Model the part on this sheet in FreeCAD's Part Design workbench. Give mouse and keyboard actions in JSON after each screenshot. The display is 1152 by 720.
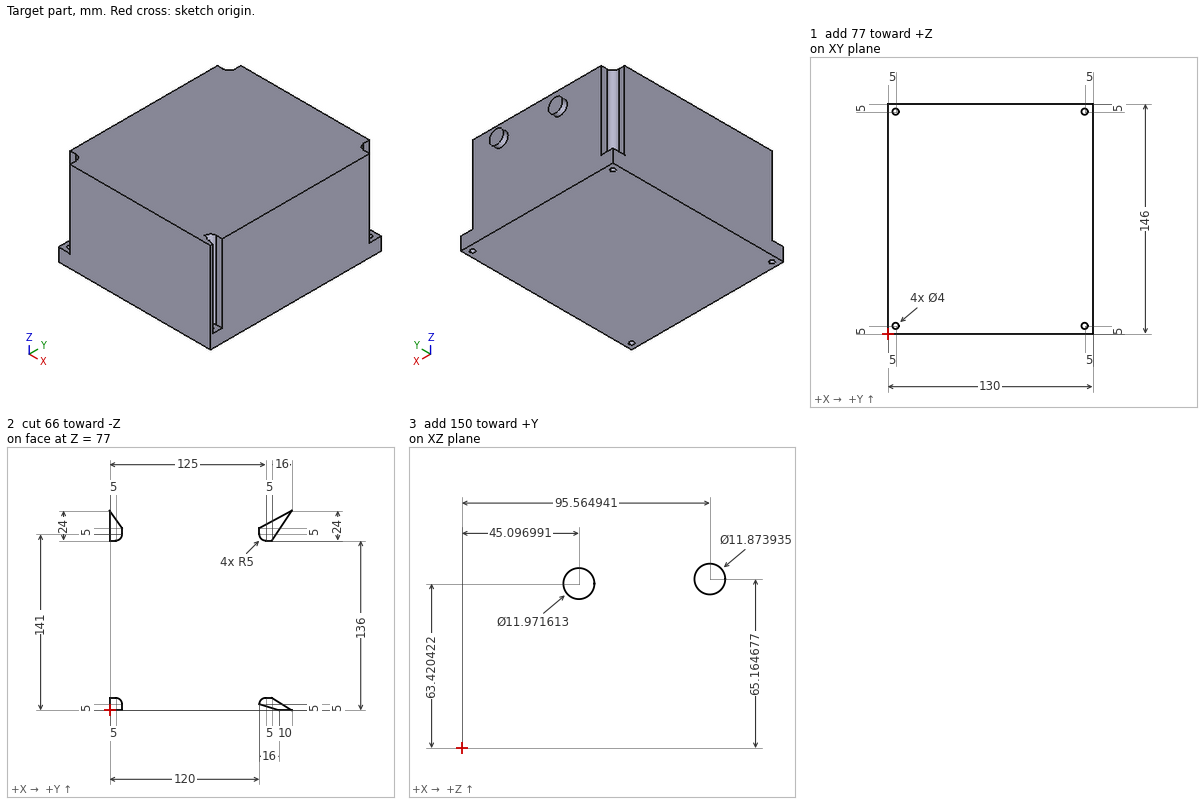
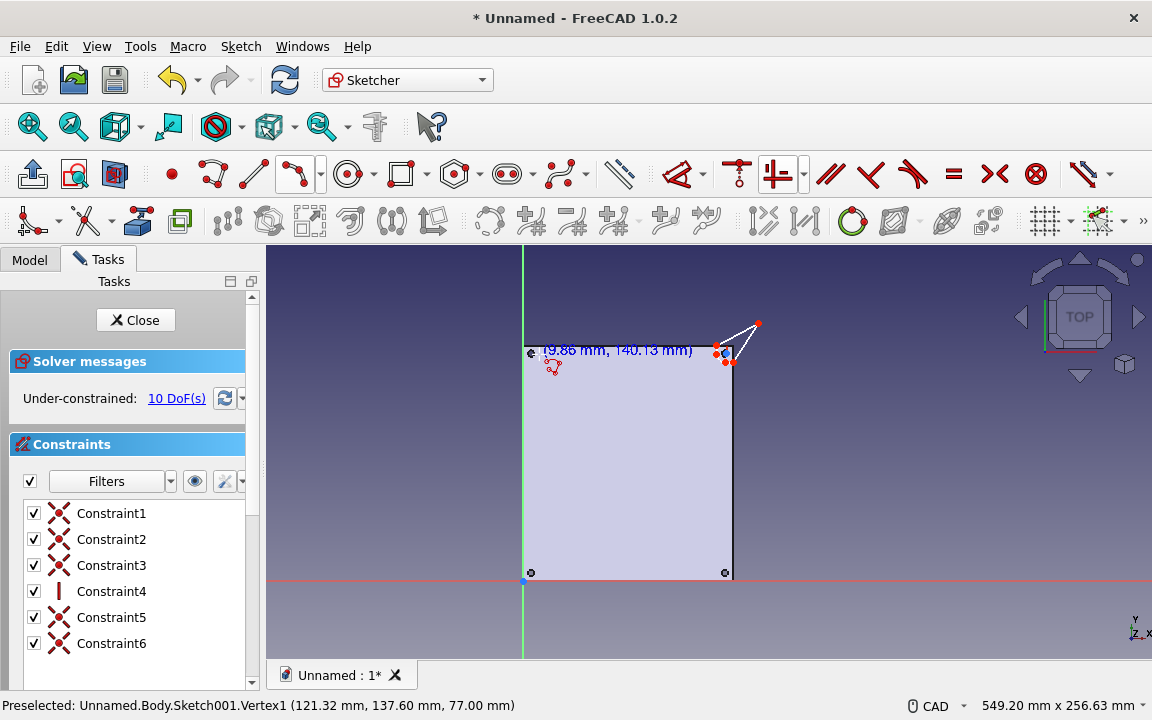
{"action": "scroll", "coordinate": [539, 346], "scroll_direction": "up", "scroll_amount": 4}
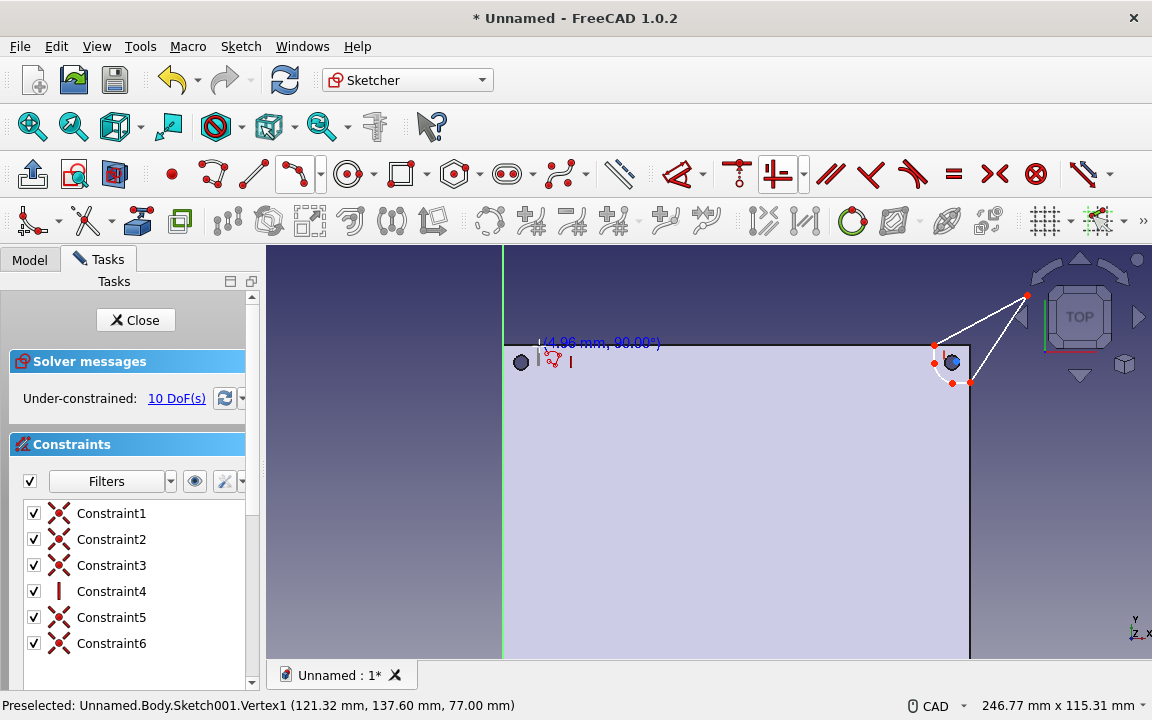
{"action": "left_click", "coordinate": [539, 345]}
{"action": "left_click", "coordinate": [503, 294]}
{"action": "left_click", "coordinate": [512, 381]}
{"action": "left_click", "coordinate": [521, 381]}
{"action": "right_click", "coordinate": [521, 381]}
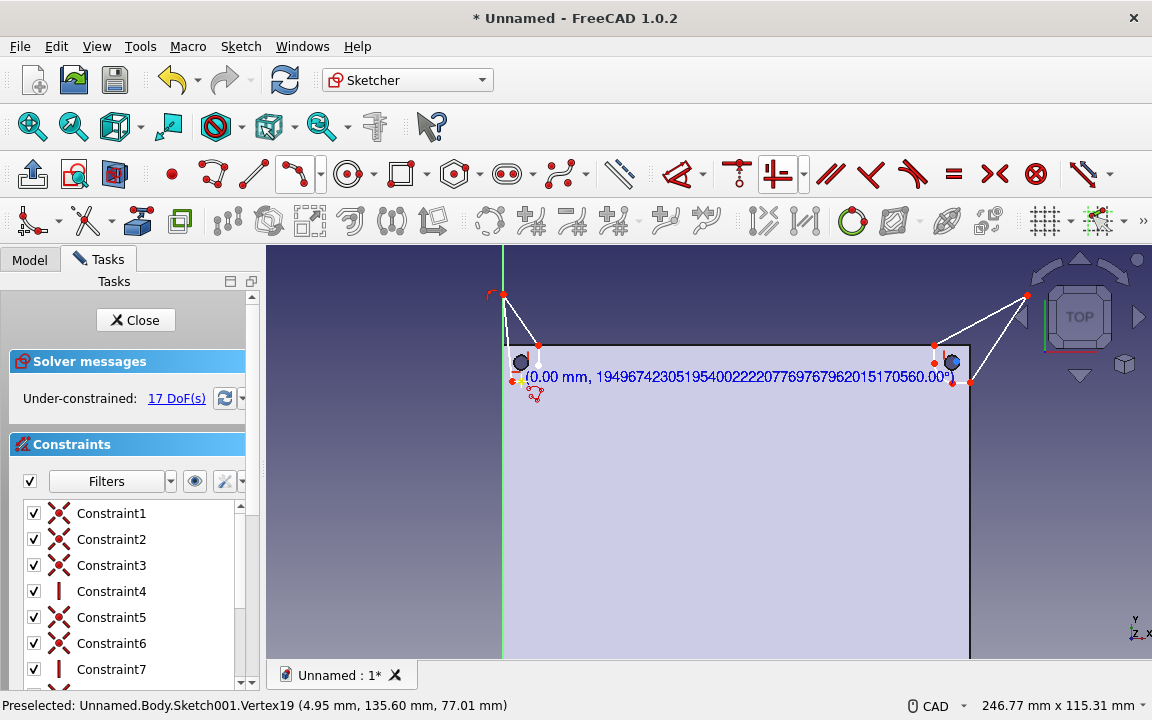
{"action": "left_click", "coordinate": [294, 174]}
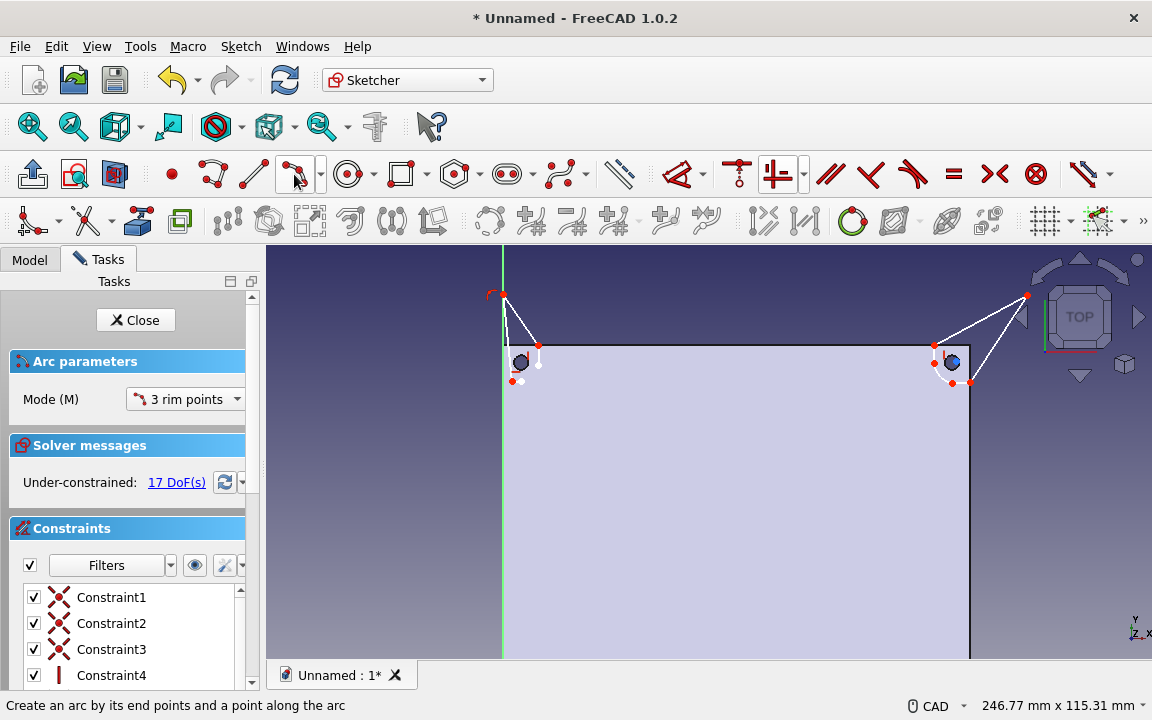
{"action": "scroll", "coordinate": [521, 381], "scroll_direction": "up", "scroll_amount": 3}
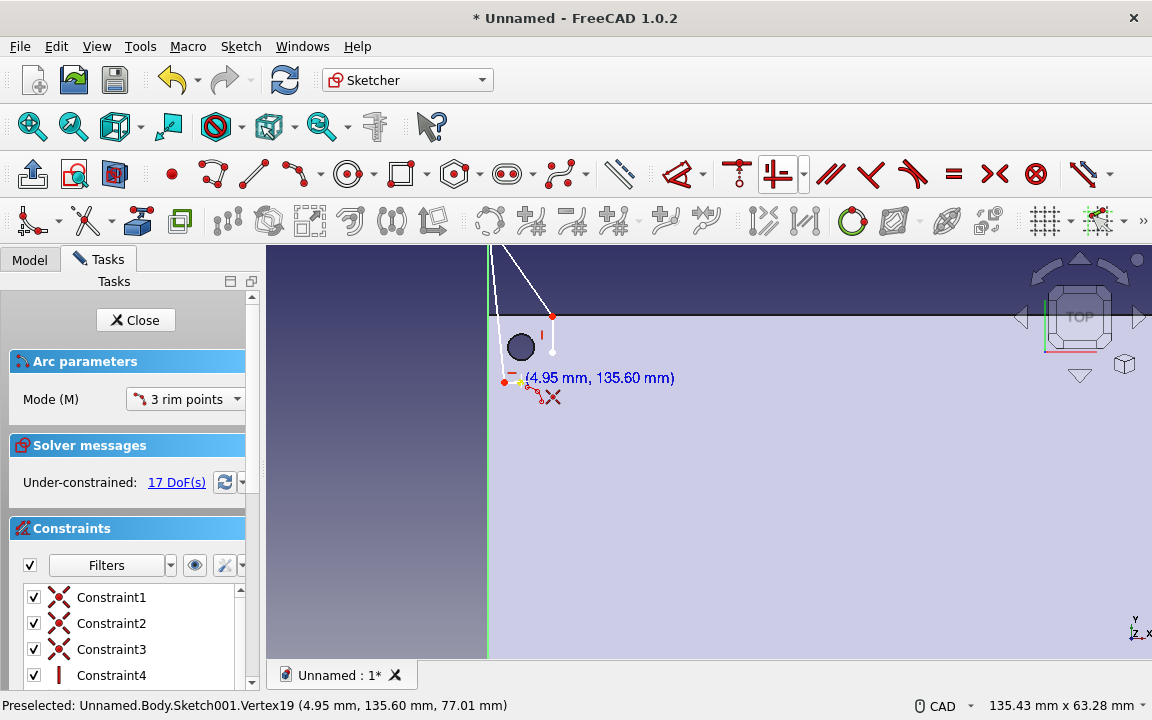
{"action": "left_click", "coordinate": [521, 383]}
{"action": "left_click", "coordinate": [553, 353]}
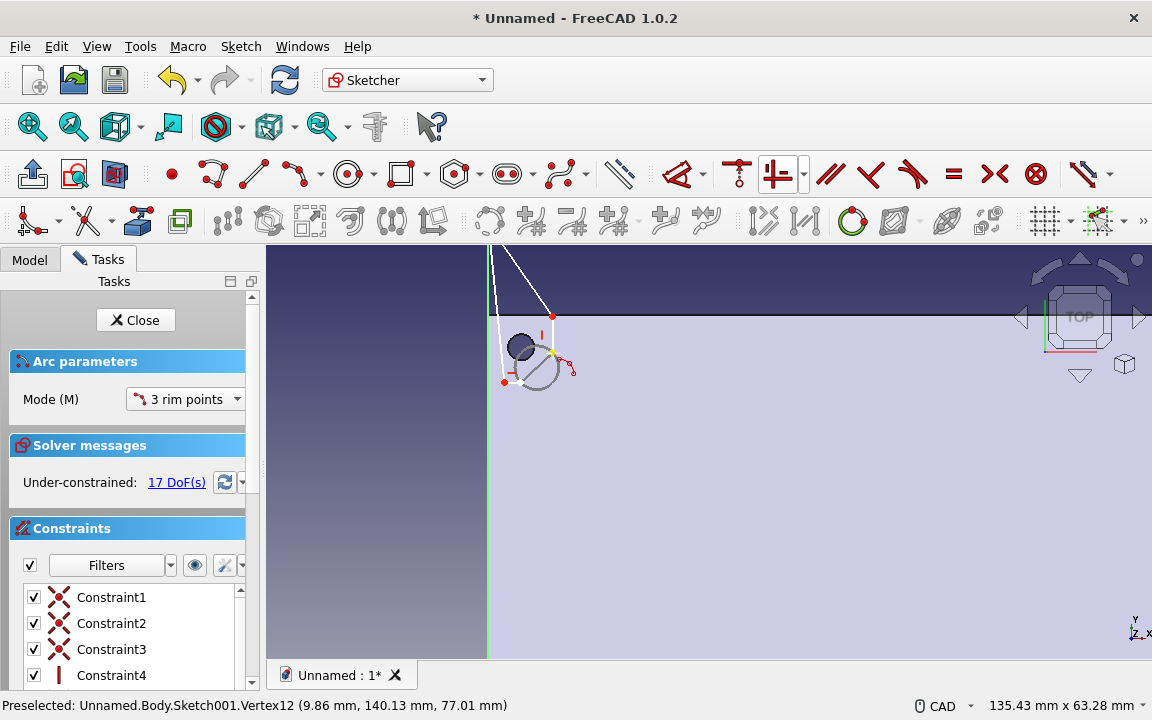
{"action": "scroll", "coordinate": [544, 370], "scroll_direction": "up", "scroll_amount": 3}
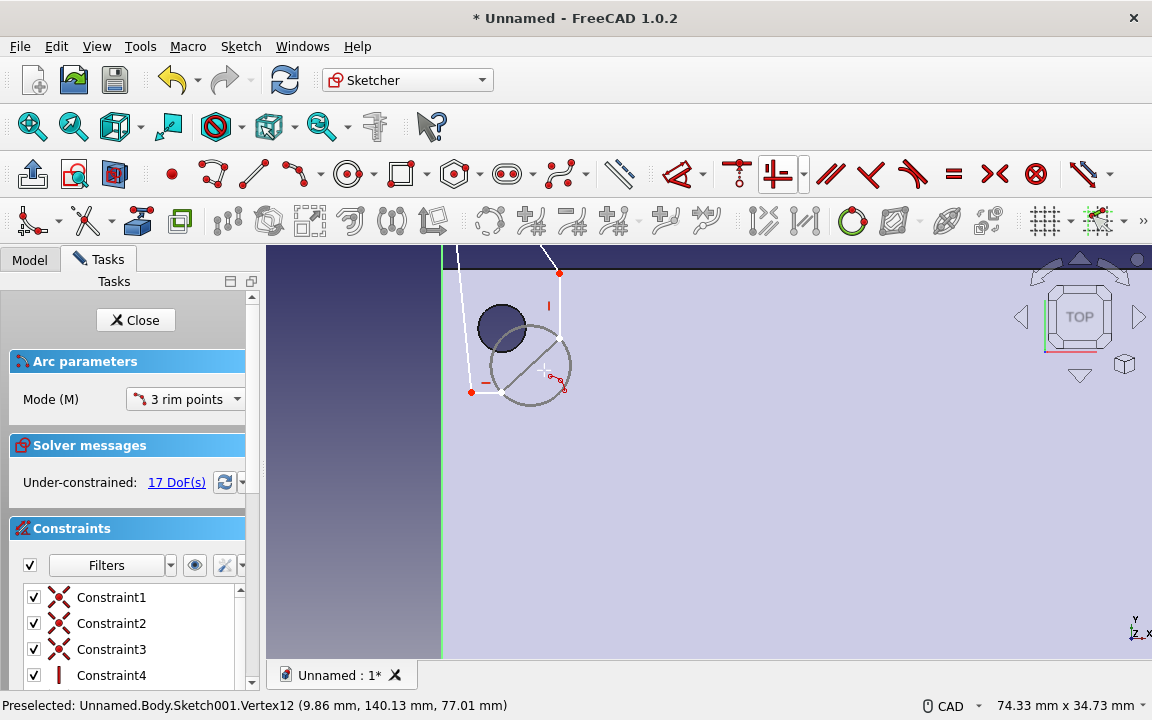
{"action": "left_click", "coordinate": [544, 370]}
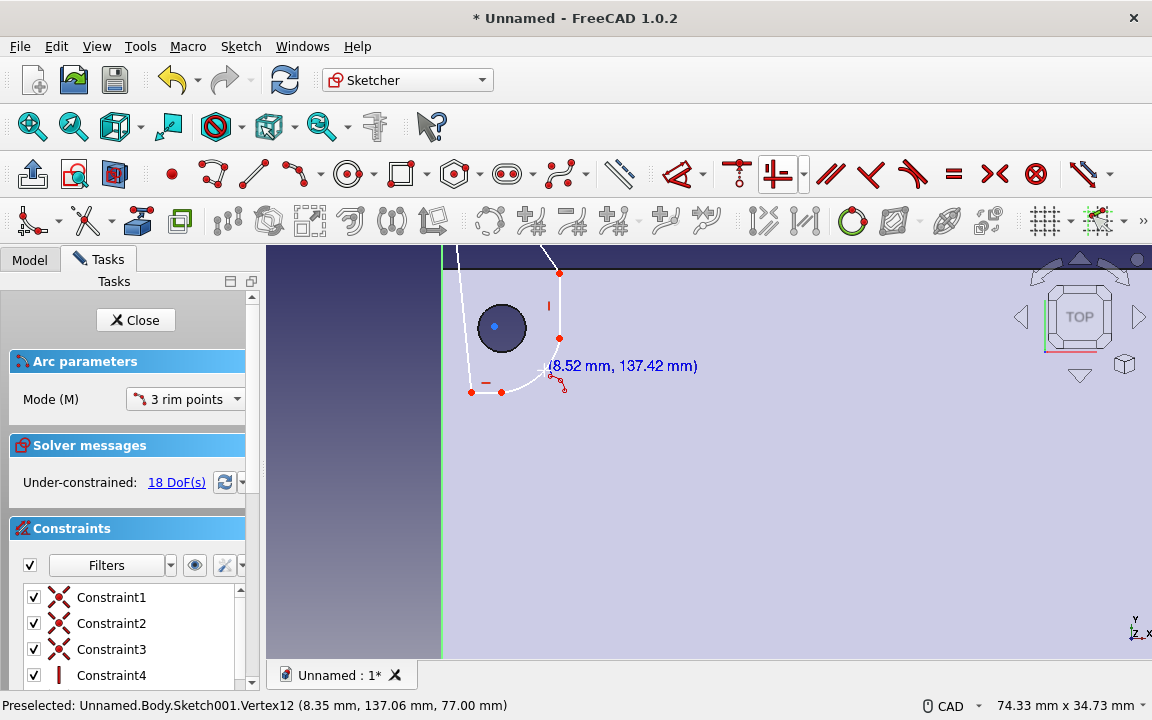
{"action": "left_click", "coordinate": [213, 174]}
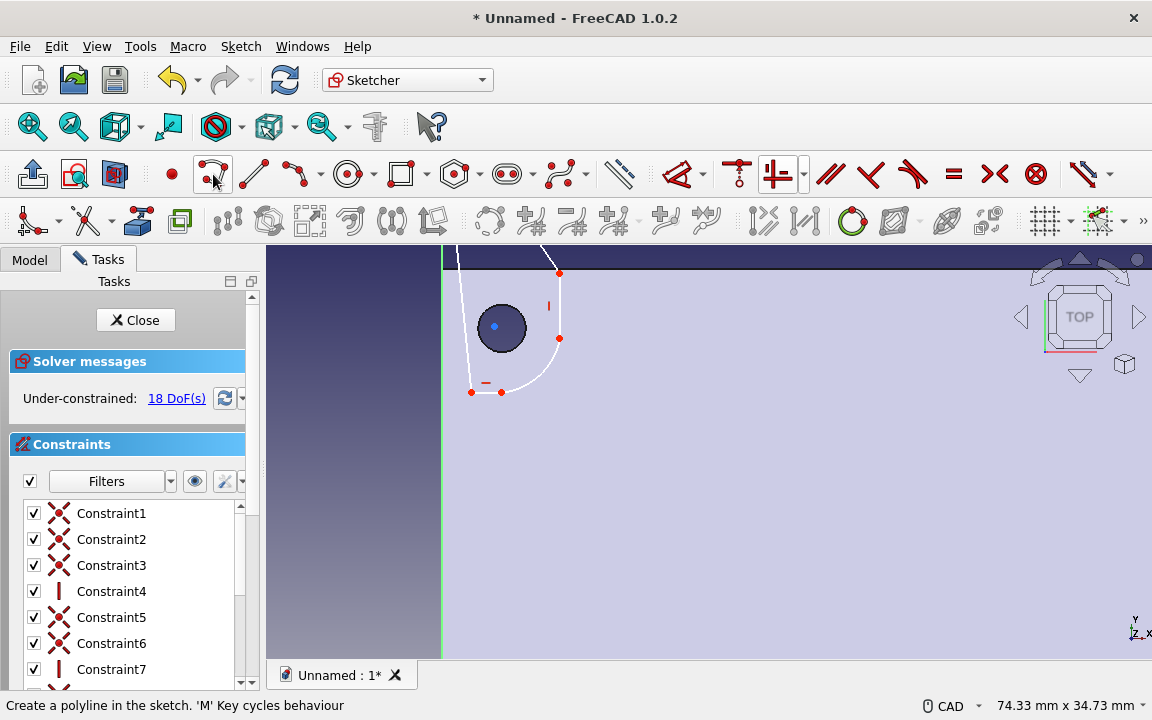
{"action": "scroll", "coordinate": [535, 358], "scroll_direction": "down", "scroll_amount": 10}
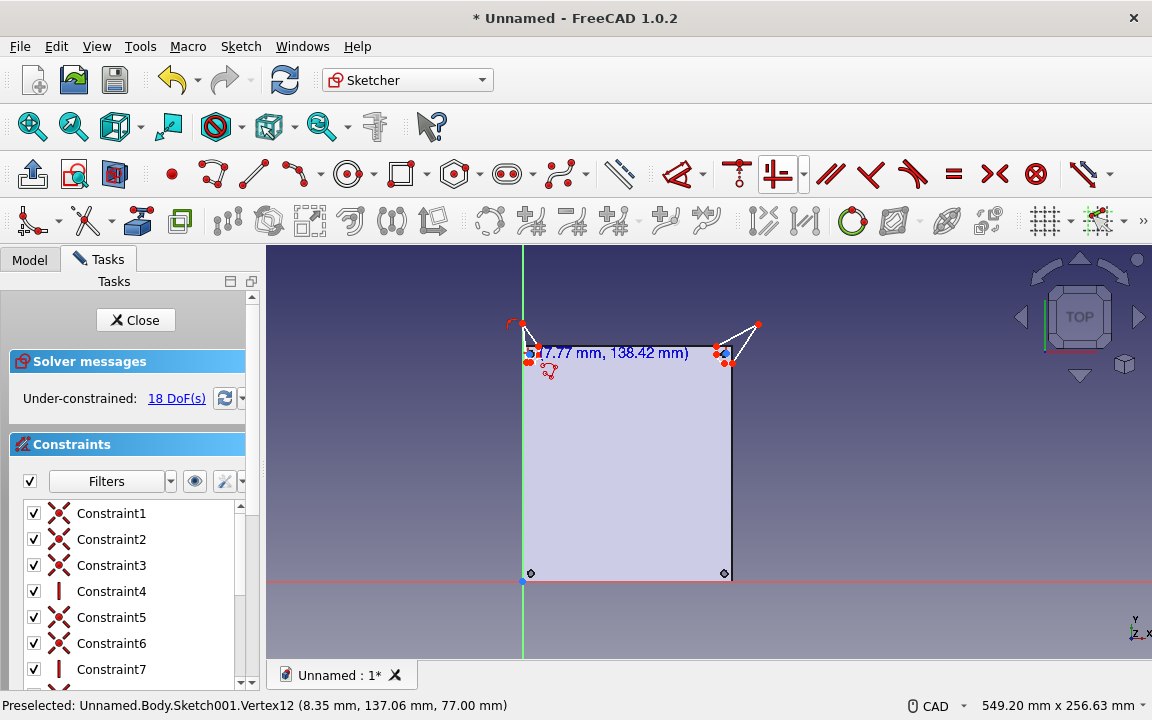
{"action": "scroll", "coordinate": [531, 566], "scroll_direction": "up", "scroll_amount": 4}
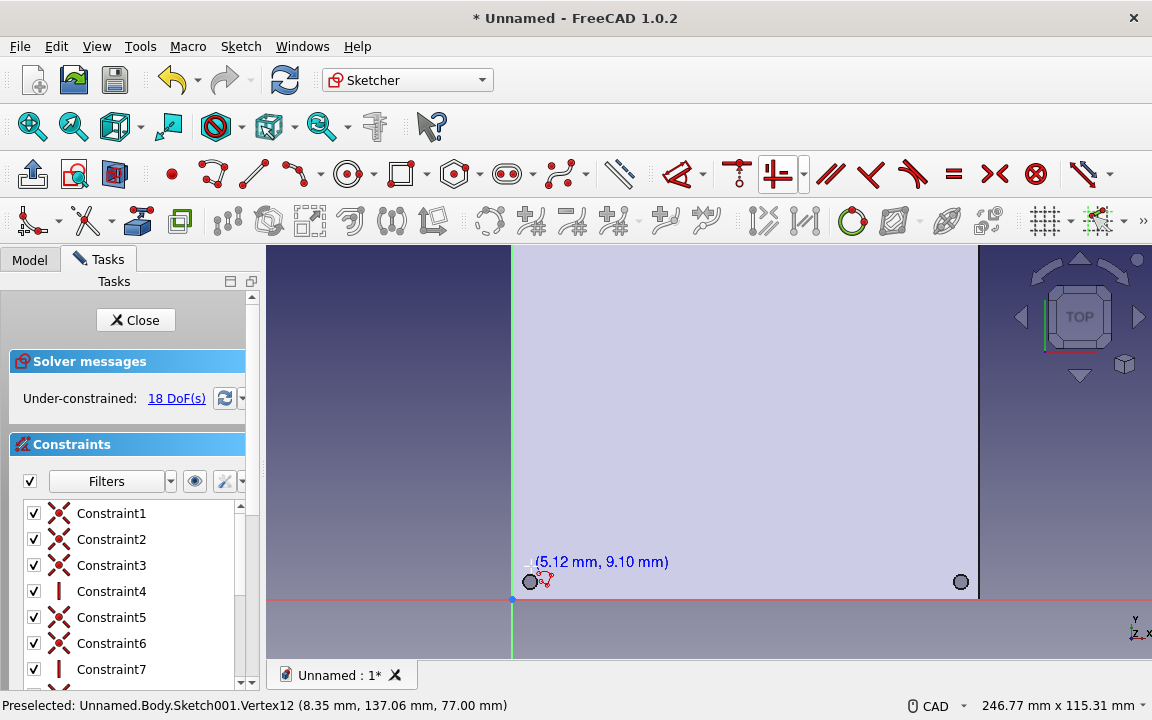
{"action": "left_click", "coordinate": [530, 564]}
{"action": "left_click", "coordinate": [512, 564]}
{"action": "left_click", "coordinate": [512, 600]}
{"action": "left_click", "coordinate": [548, 591]}
{"action": "left_click", "coordinate": [548, 582]}
{"action": "right_click", "coordinate": [548, 582]}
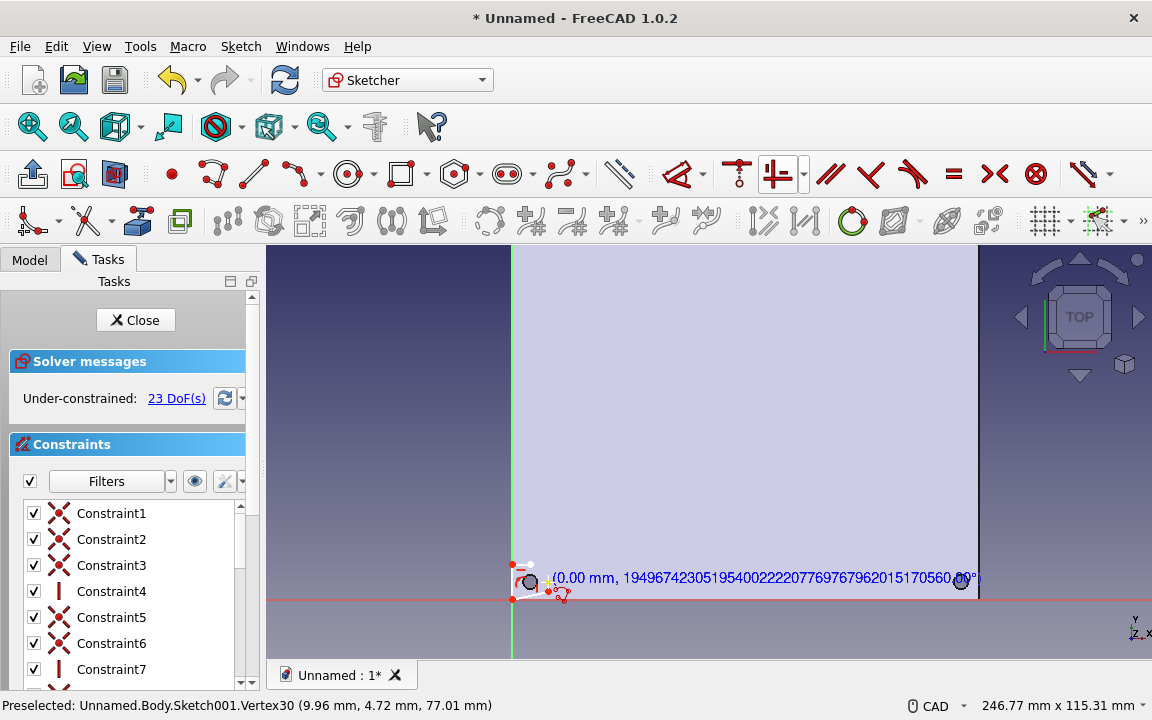
{"action": "left_click", "coordinate": [294, 174]}